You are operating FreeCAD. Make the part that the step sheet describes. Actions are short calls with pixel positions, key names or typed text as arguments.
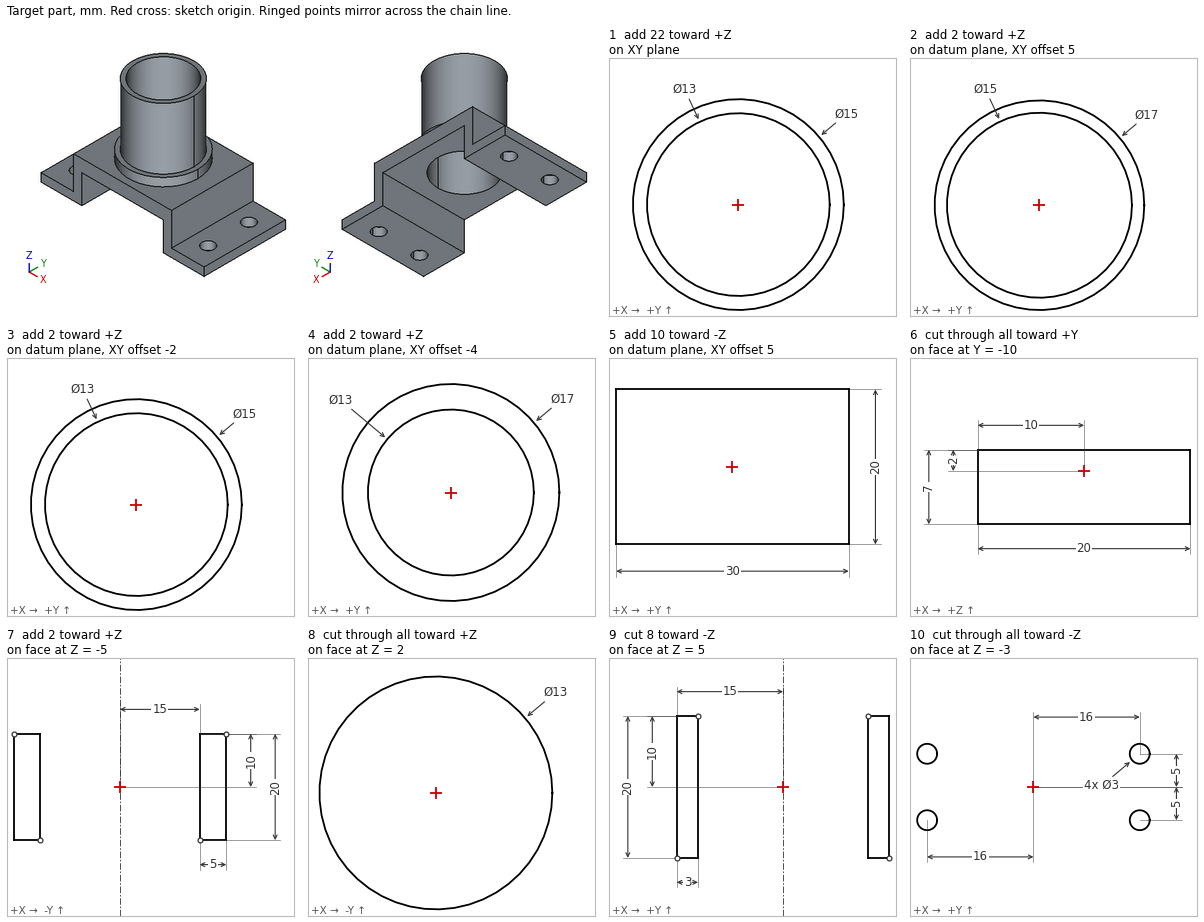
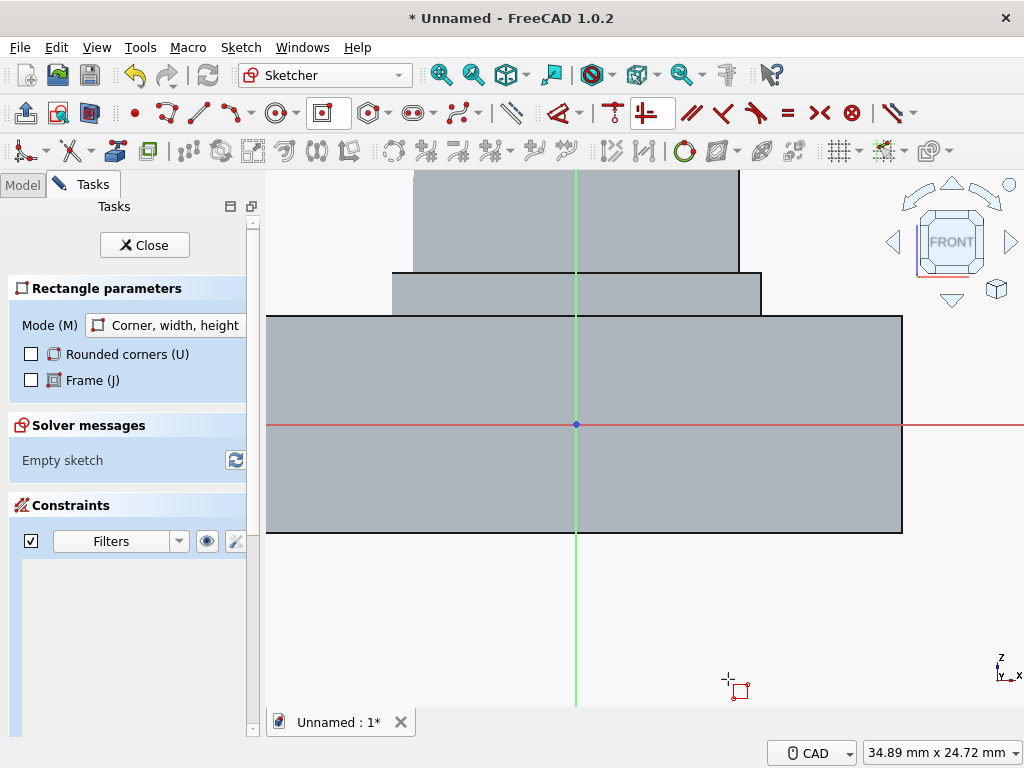
click(359, 381)
click(793, 533)
key(Escape)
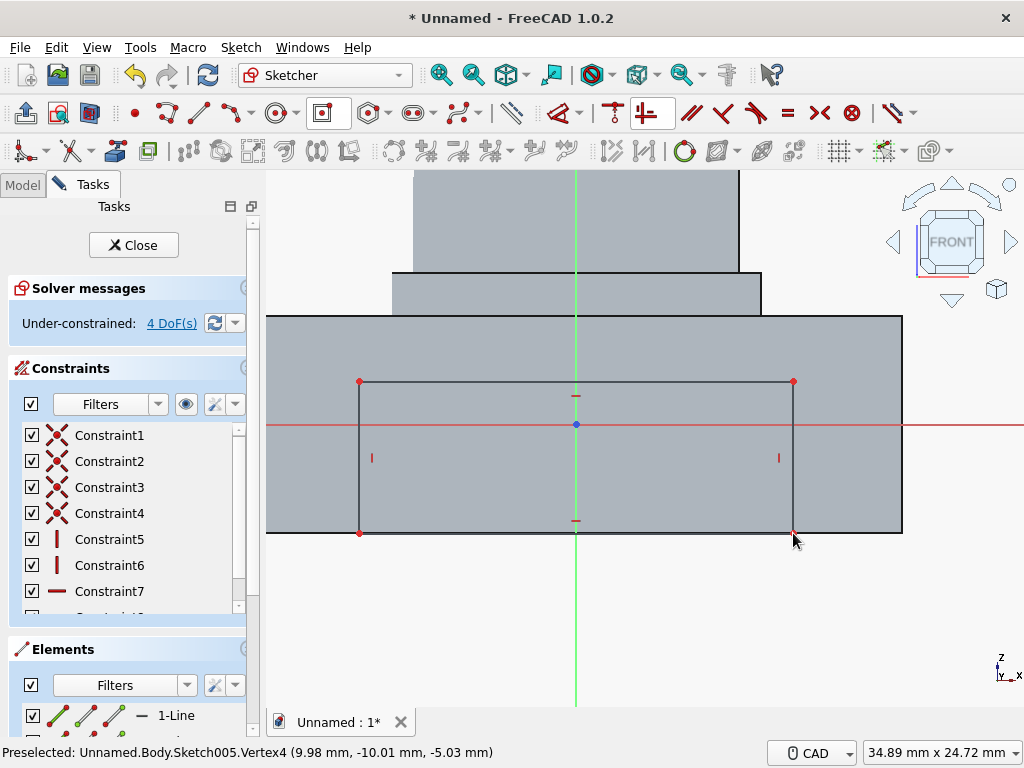
click(558, 114)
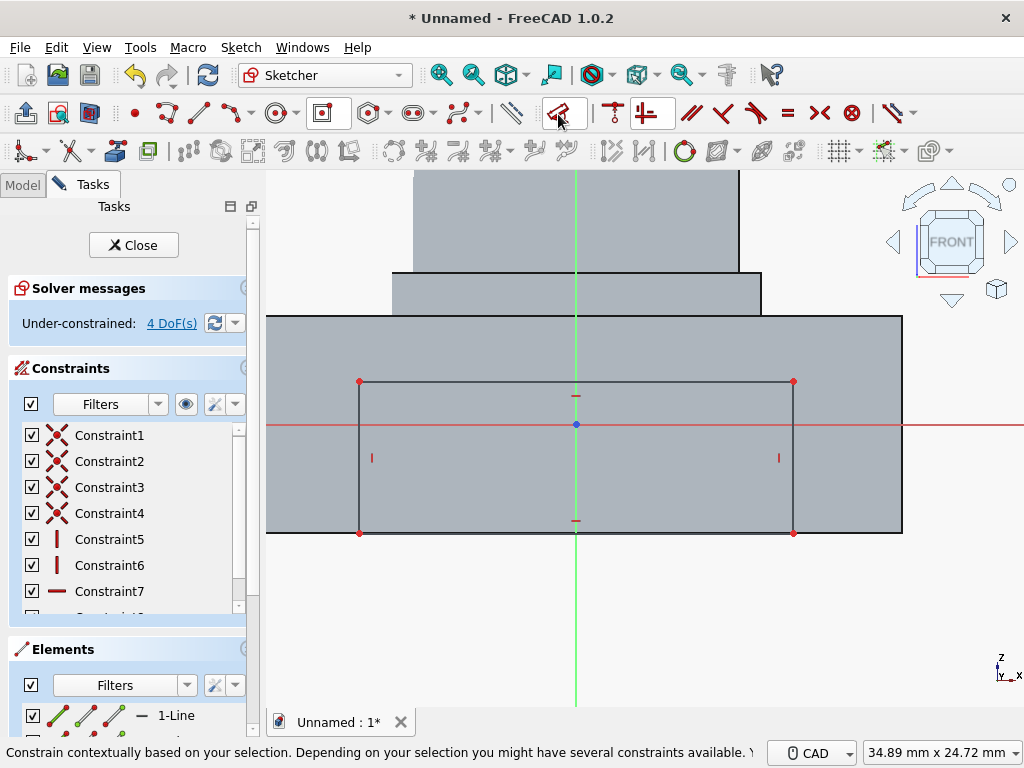
click(359, 428)
click(325, 458)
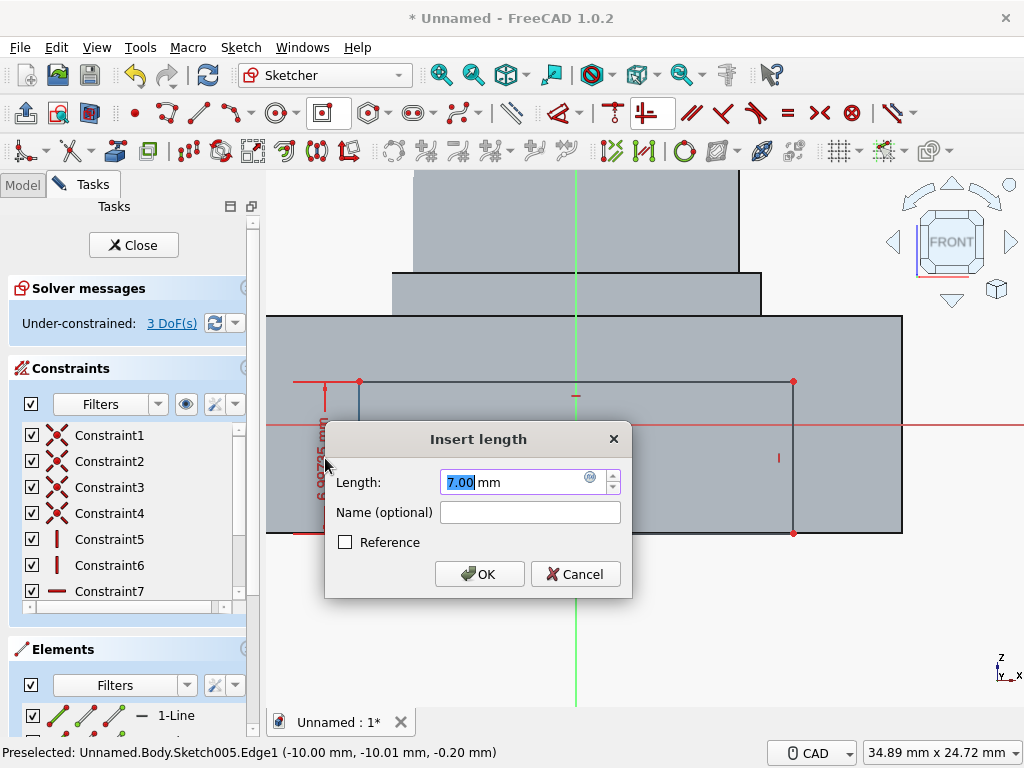
text(7)
key(Return)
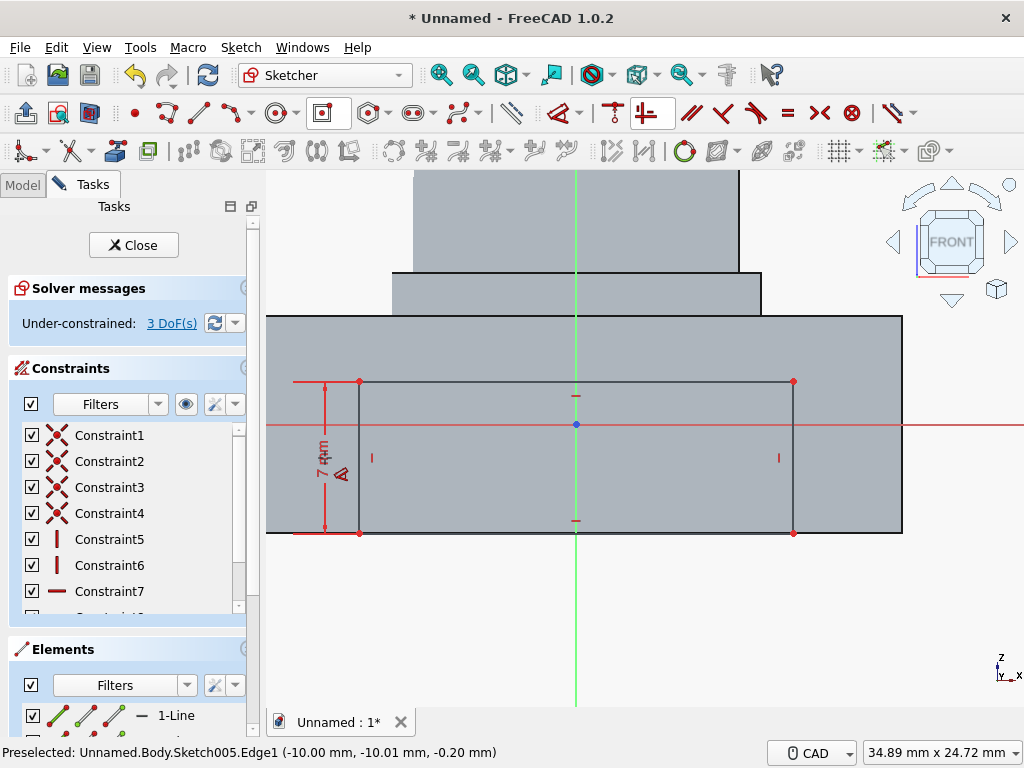
click(489, 534)
click(476, 568)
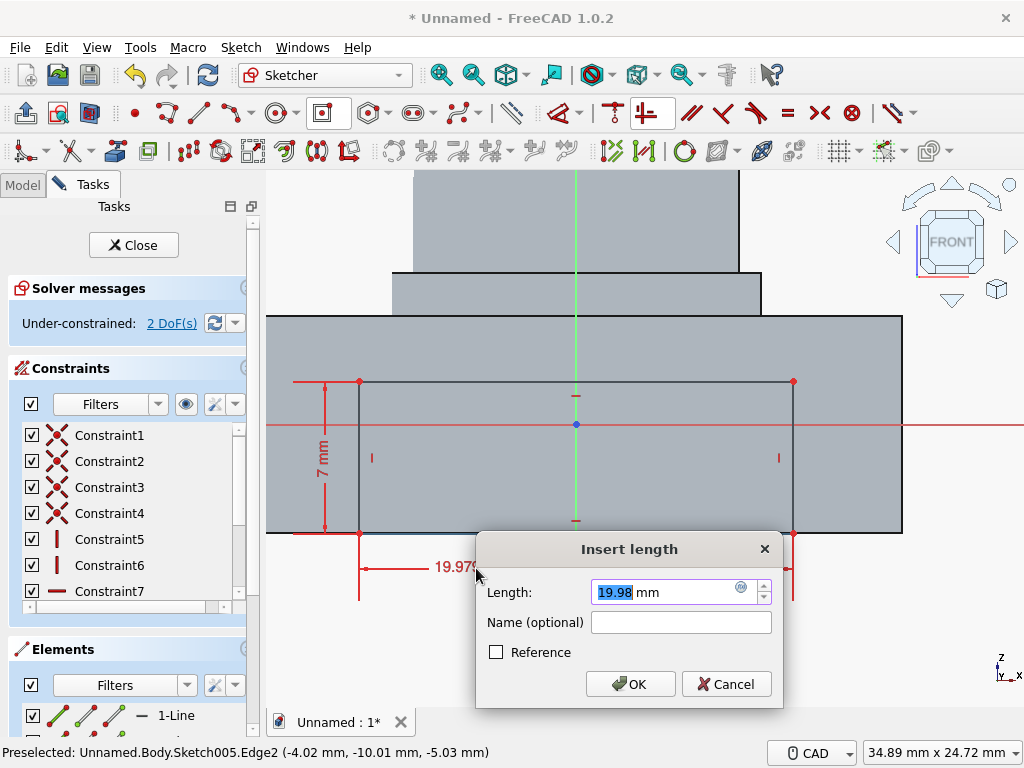
text(20)
key(Return)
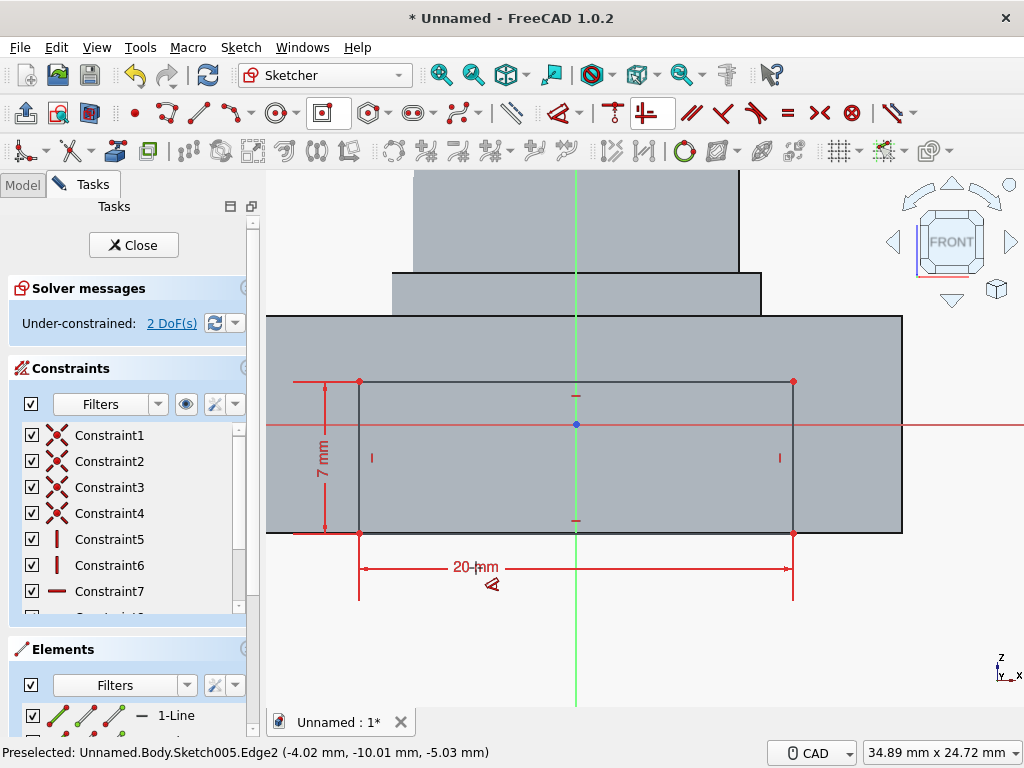
click(359, 382)
click(325, 403)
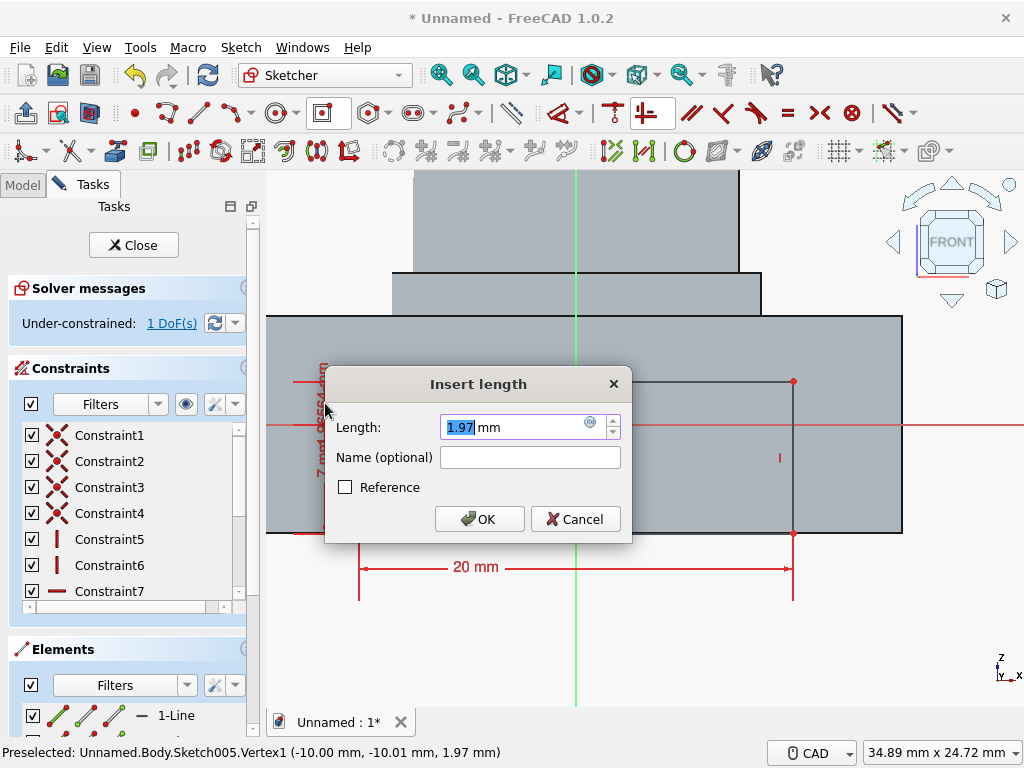
text(2)
key(Return)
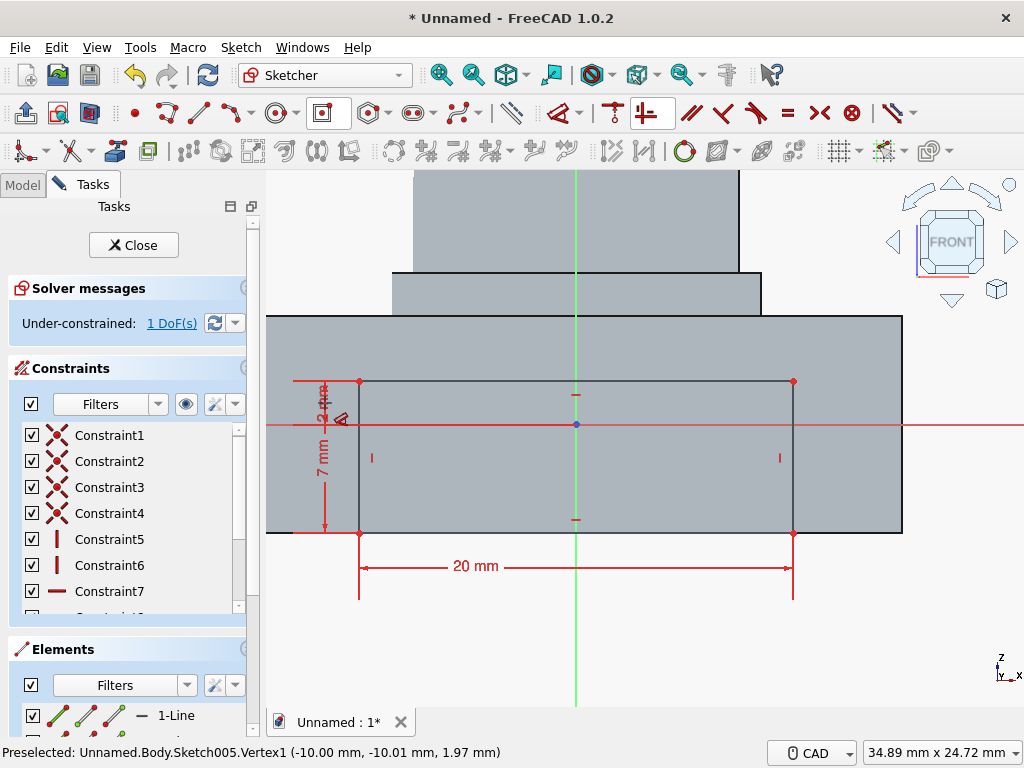
click(359, 381)
click(468, 347)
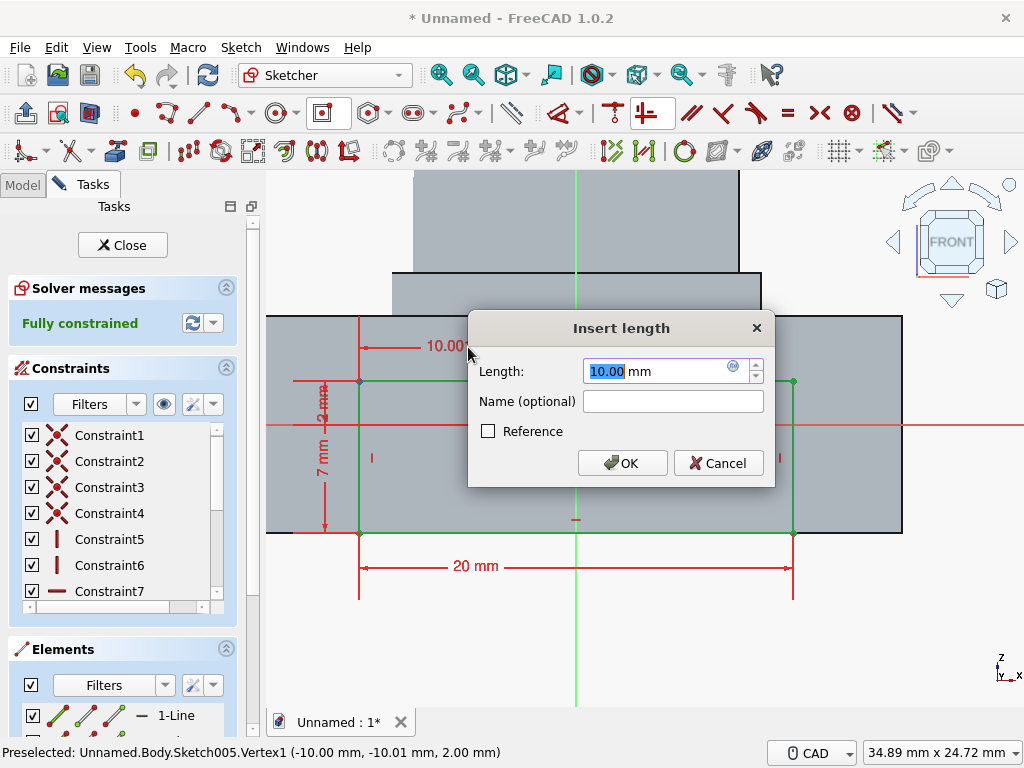
text(10)
key(Return)
key(Escape)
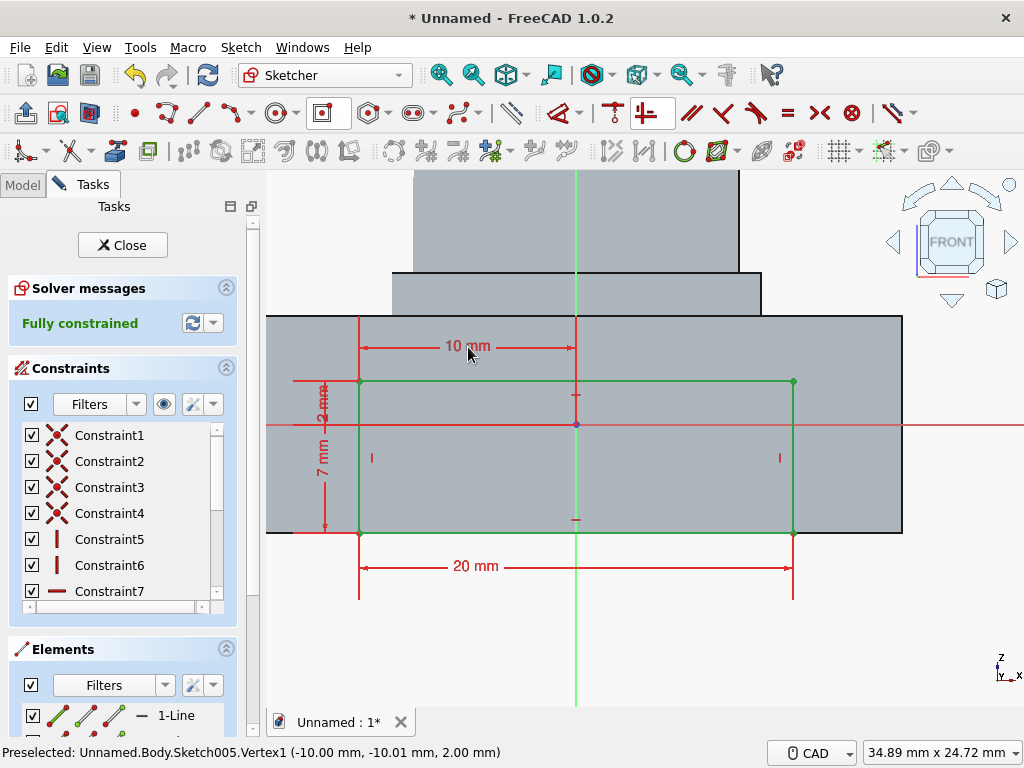
click(123, 245)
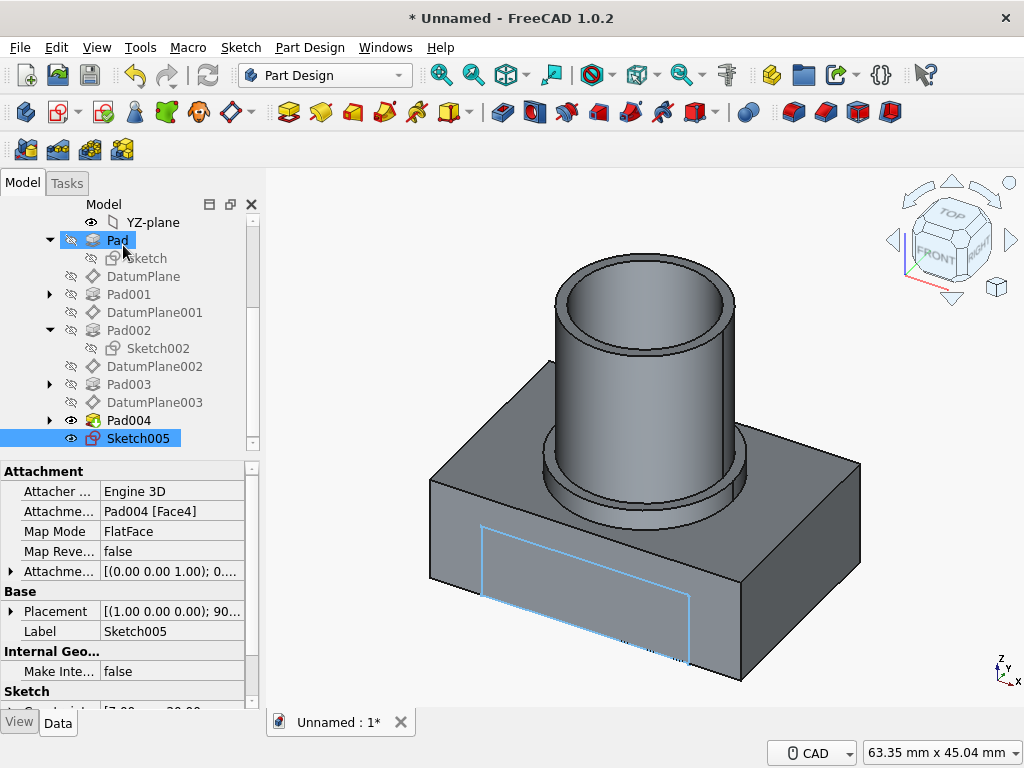
click(504, 112)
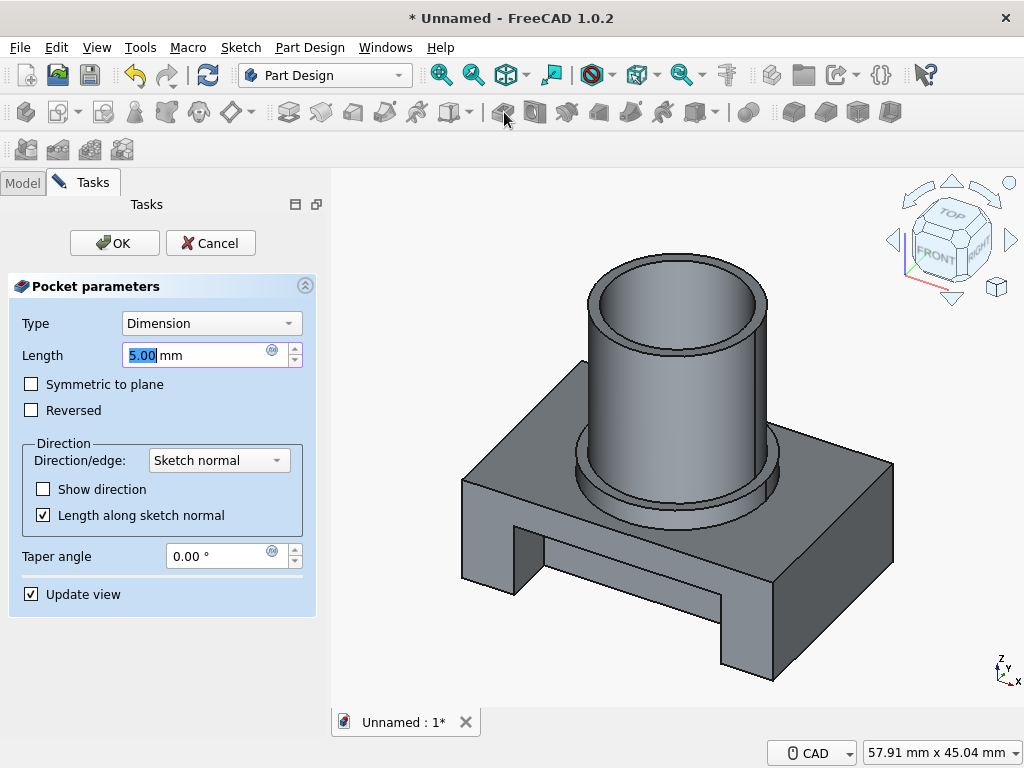
click(212, 324)